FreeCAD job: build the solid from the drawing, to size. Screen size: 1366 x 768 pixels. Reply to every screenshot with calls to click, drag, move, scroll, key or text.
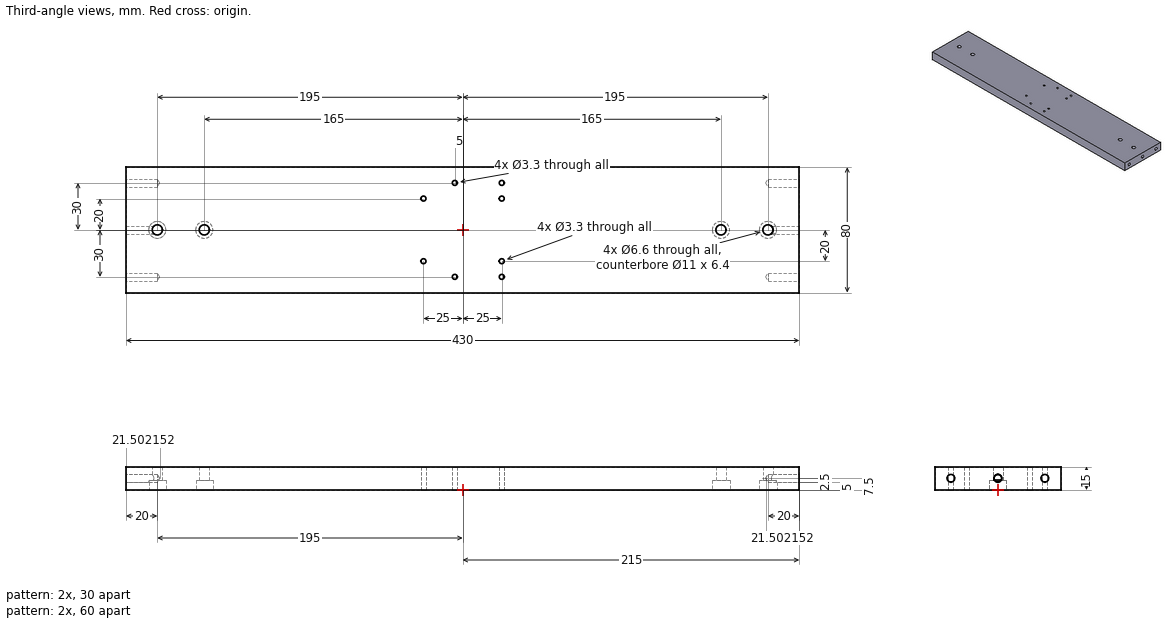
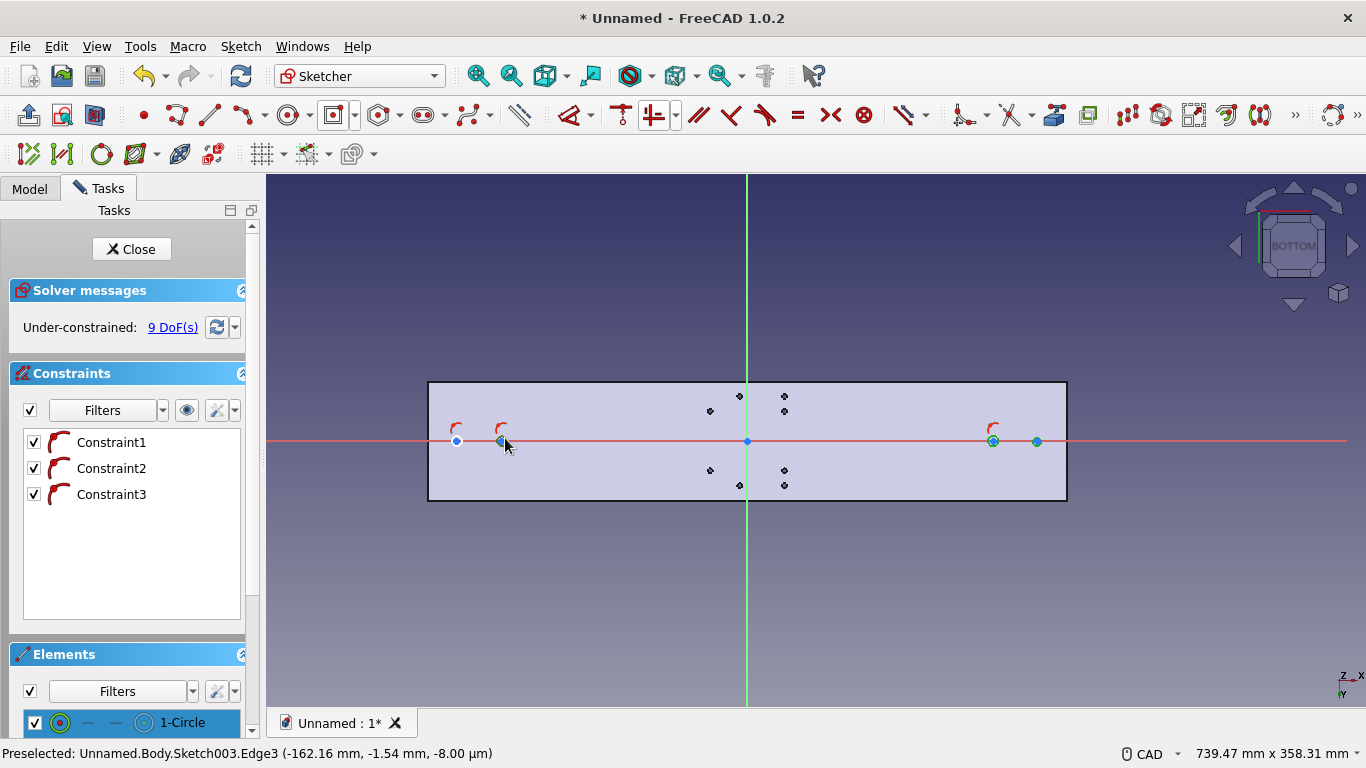
scroll(460, 438, up, 7)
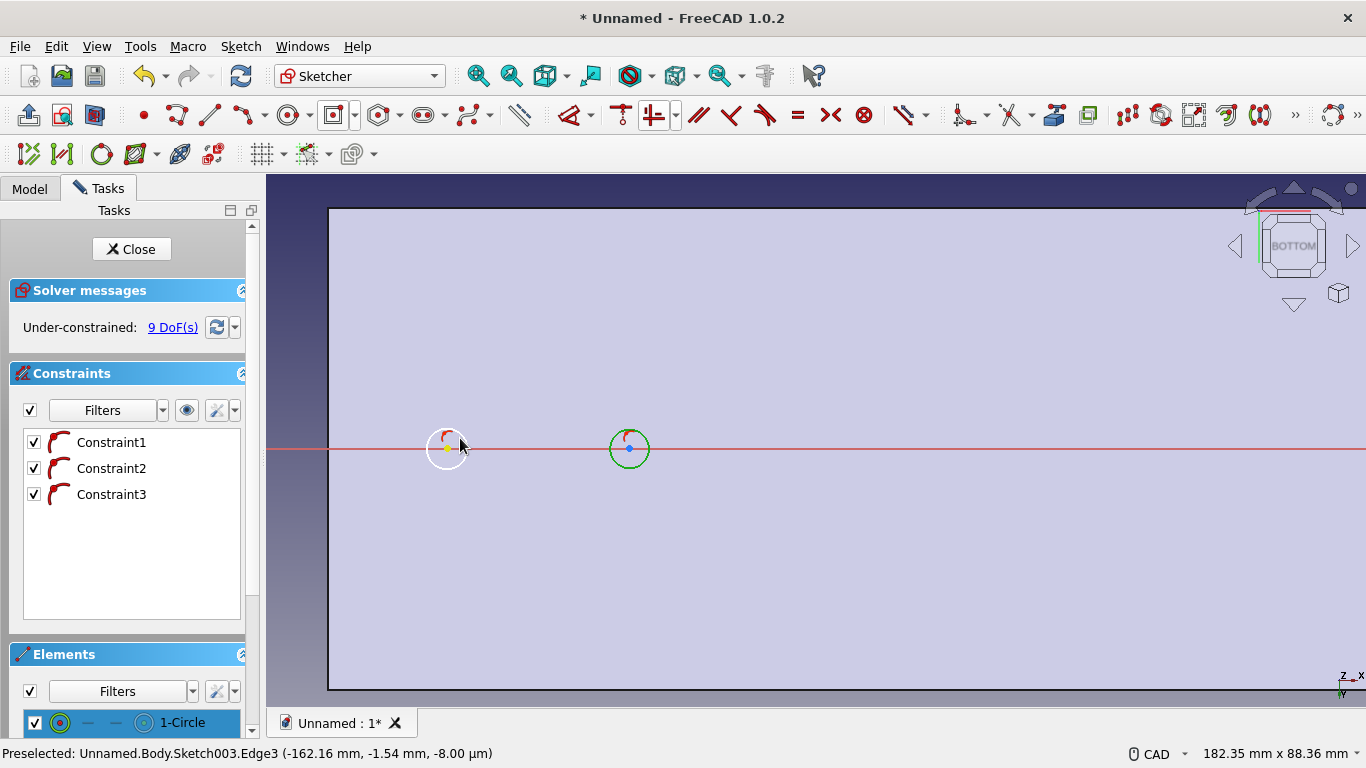
click(461, 435)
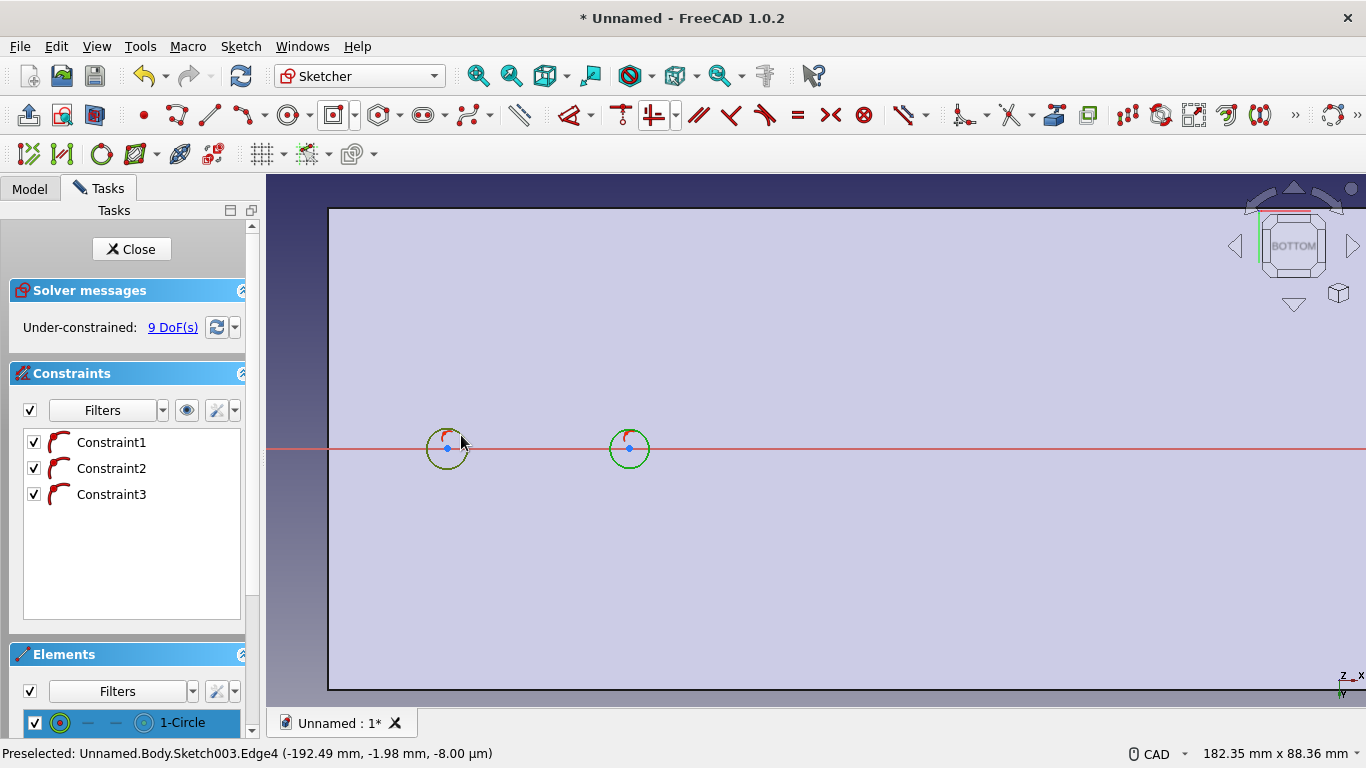
key(e)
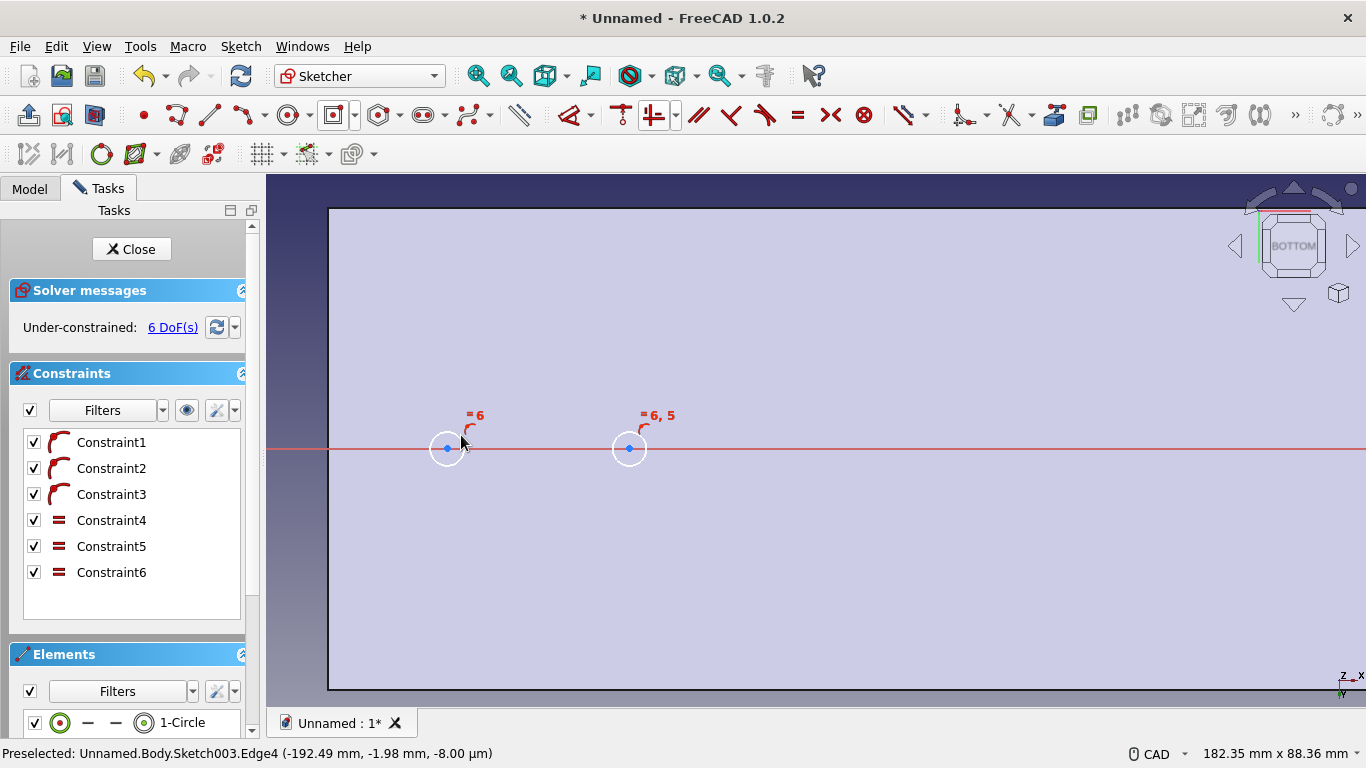
scroll(460, 438, down, 7)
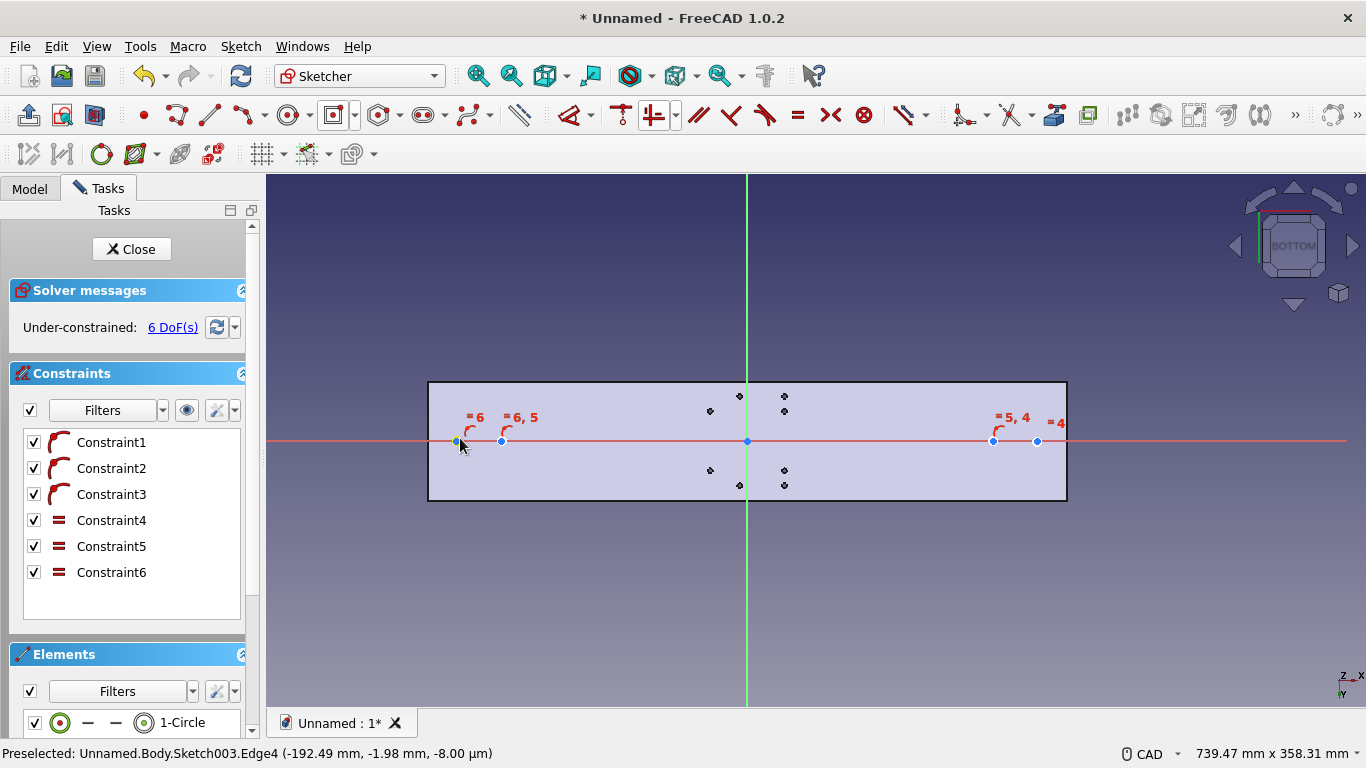
click(1037, 442)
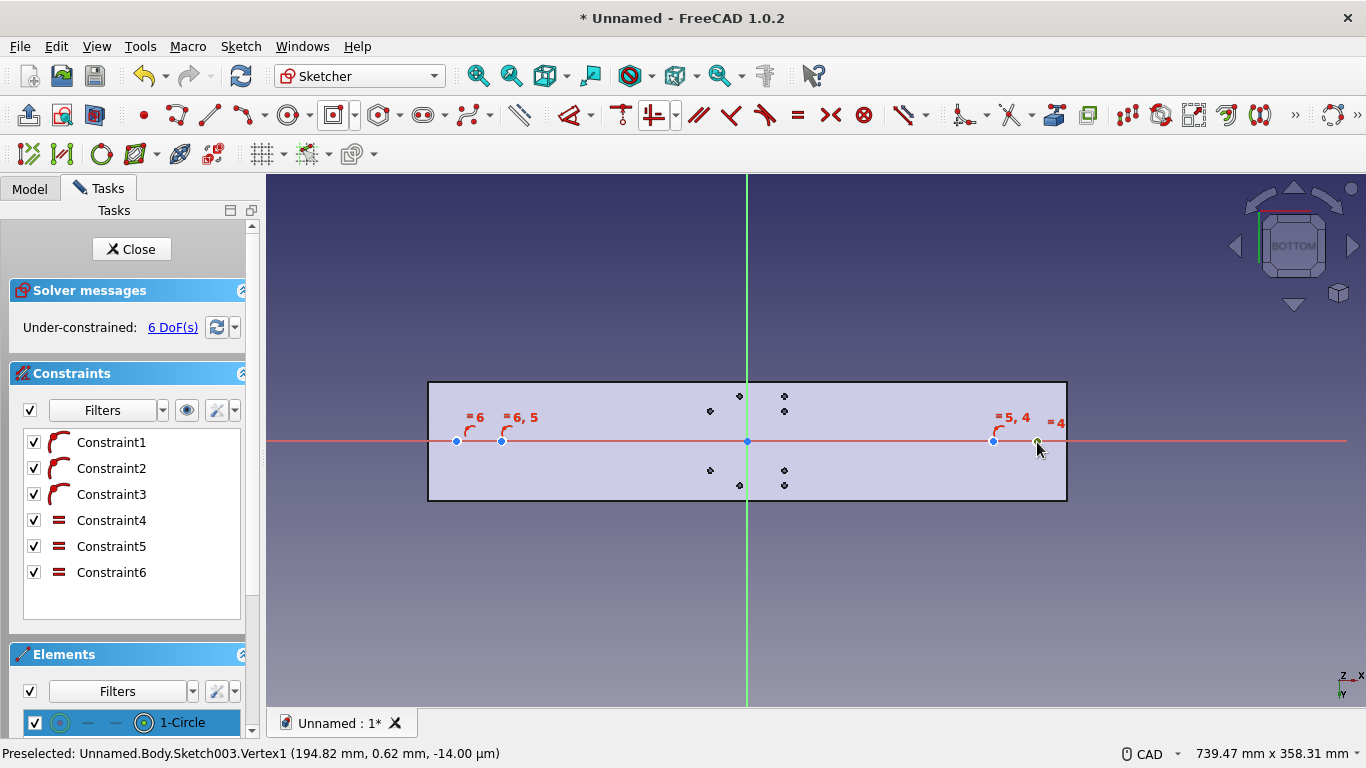
click(359, 441)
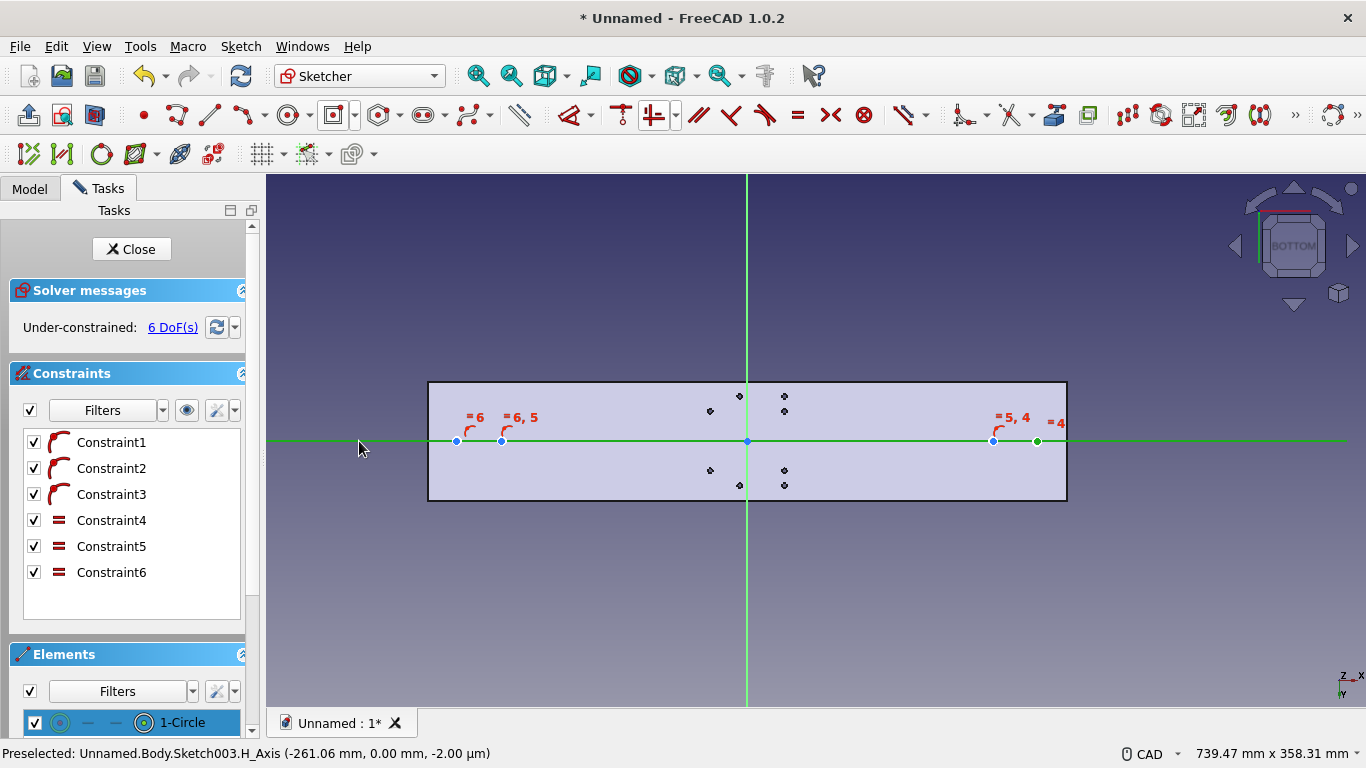
click(621, 116)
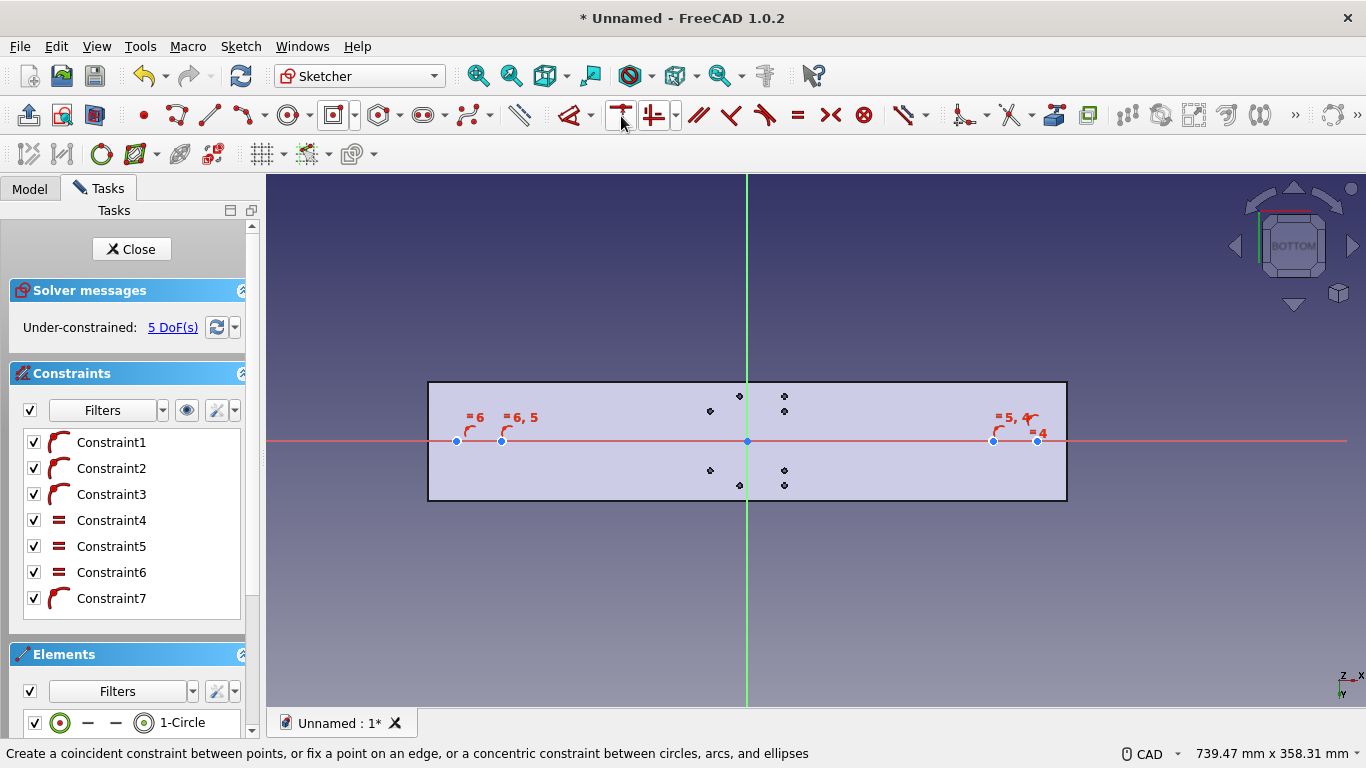
click(568, 116)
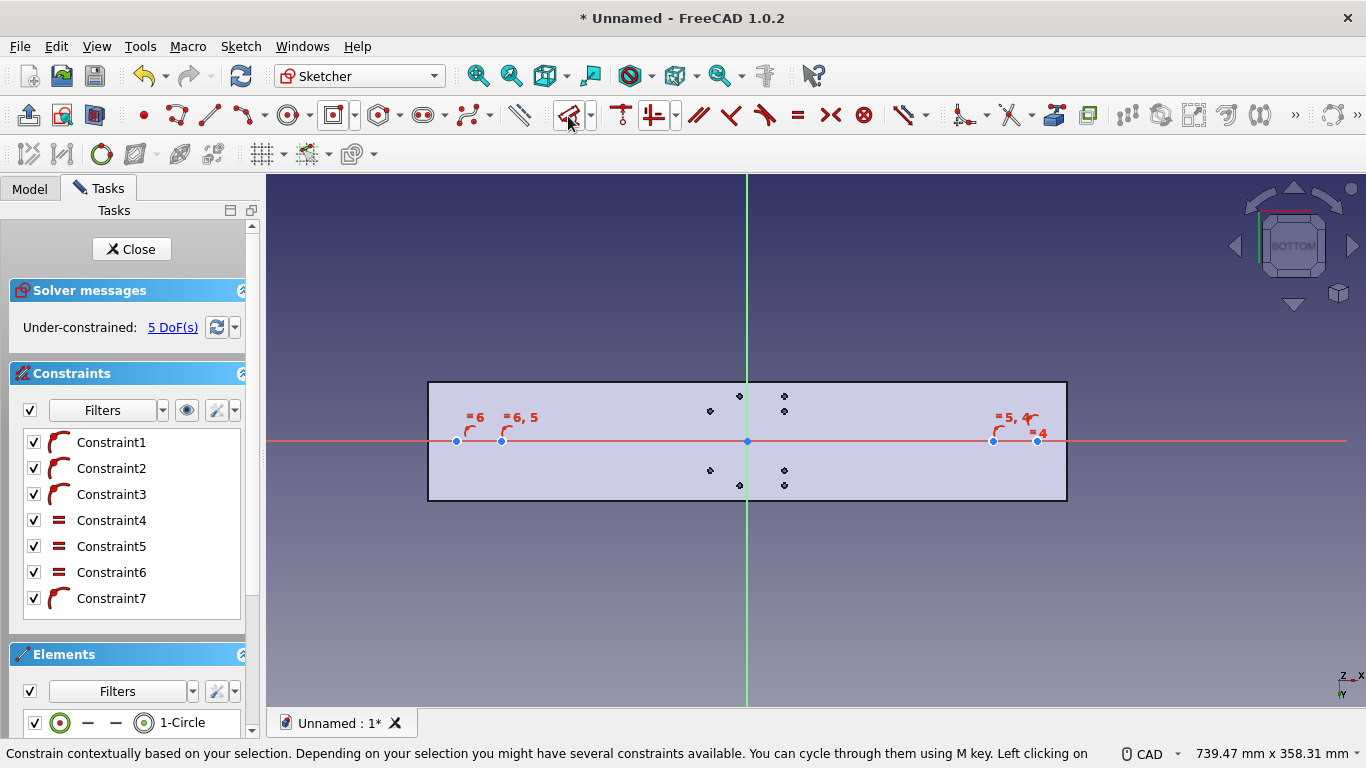
scroll(1033, 441, up, 7)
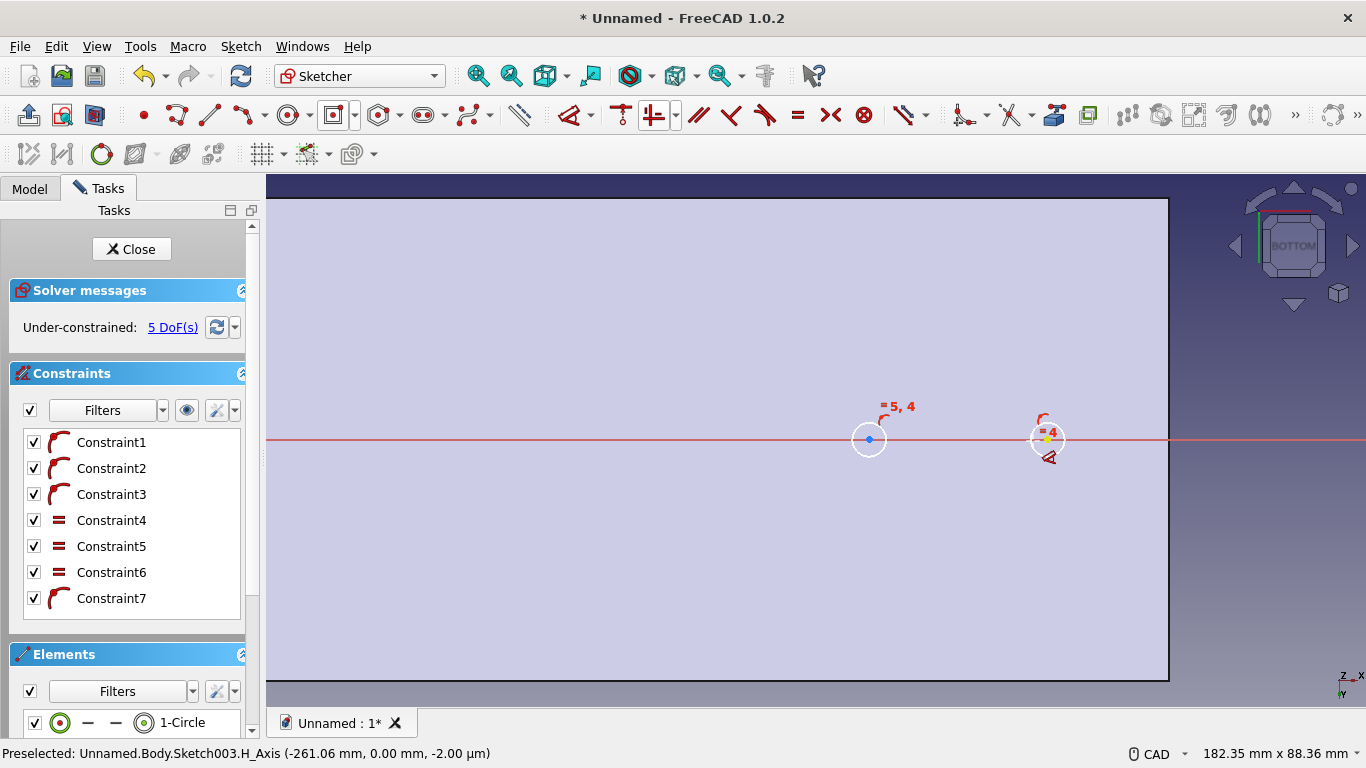
click(1031, 439)
click(1006, 414)